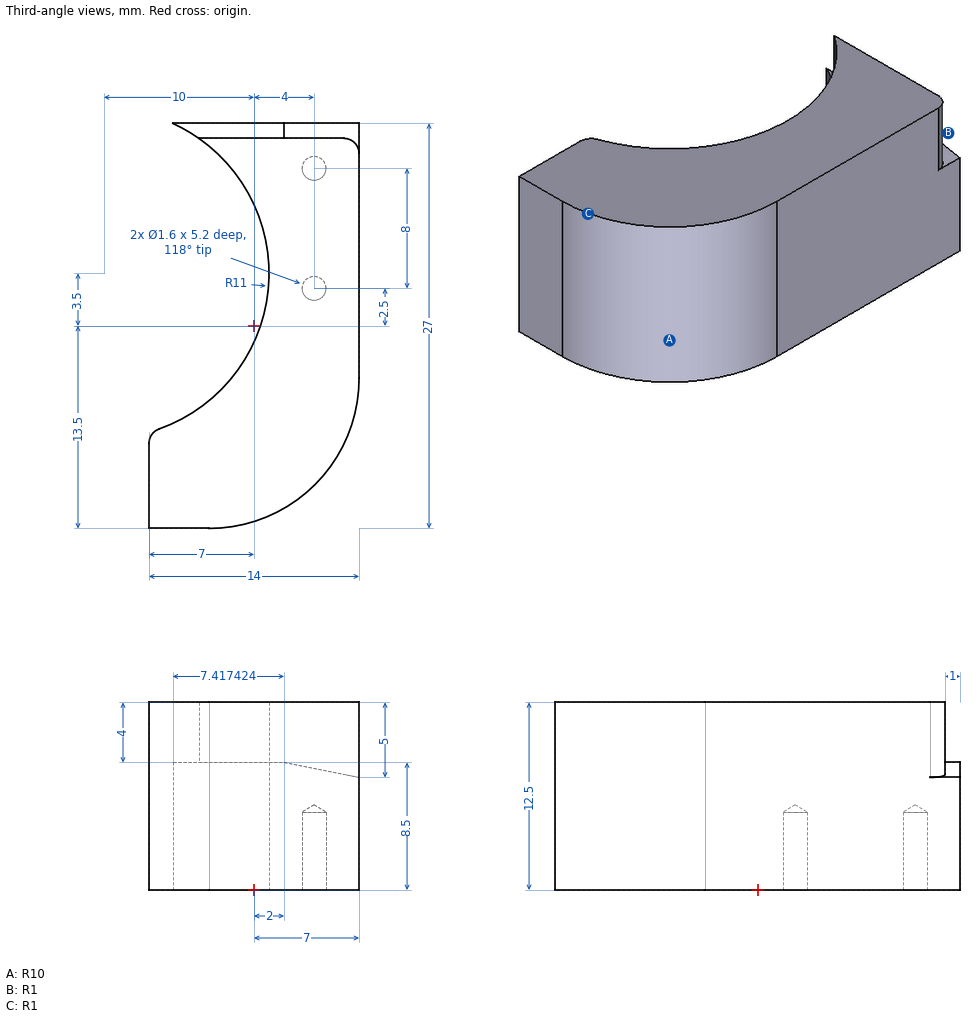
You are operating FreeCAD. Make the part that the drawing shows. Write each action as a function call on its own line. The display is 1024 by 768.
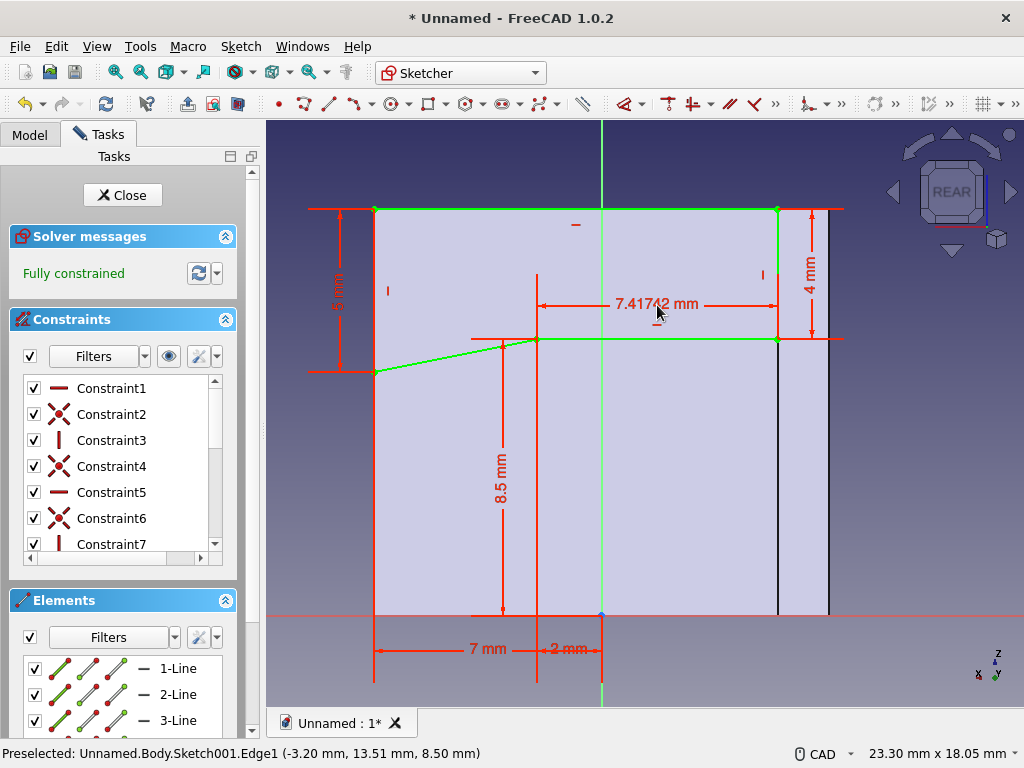
click(123, 195)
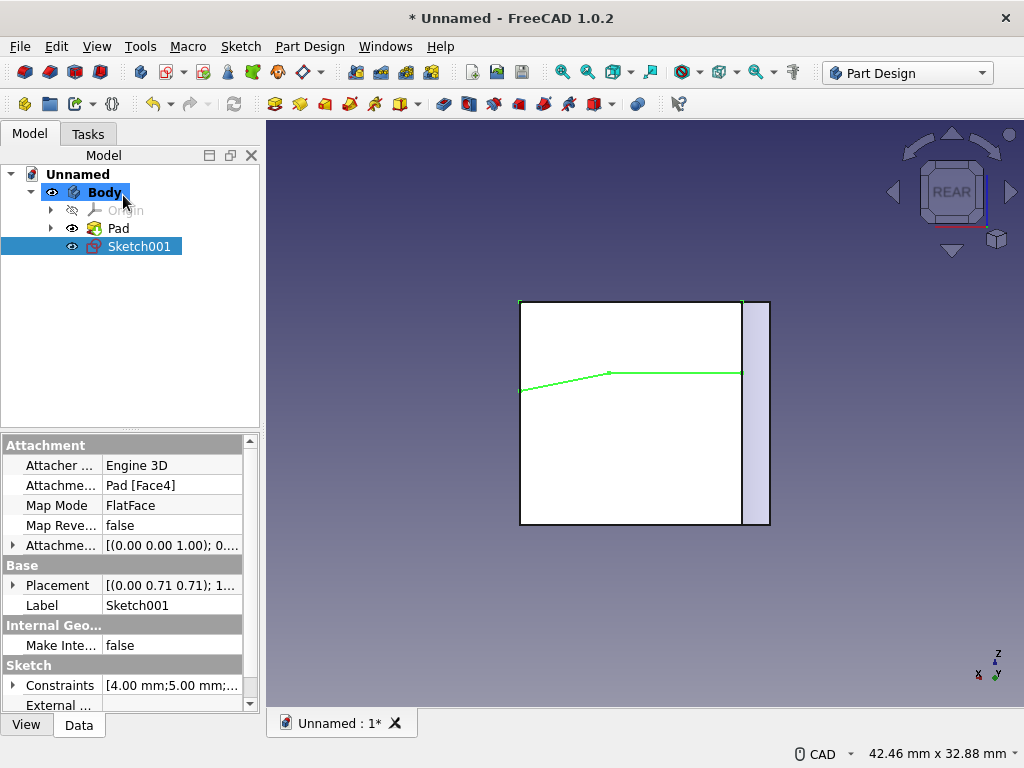
click(444, 104)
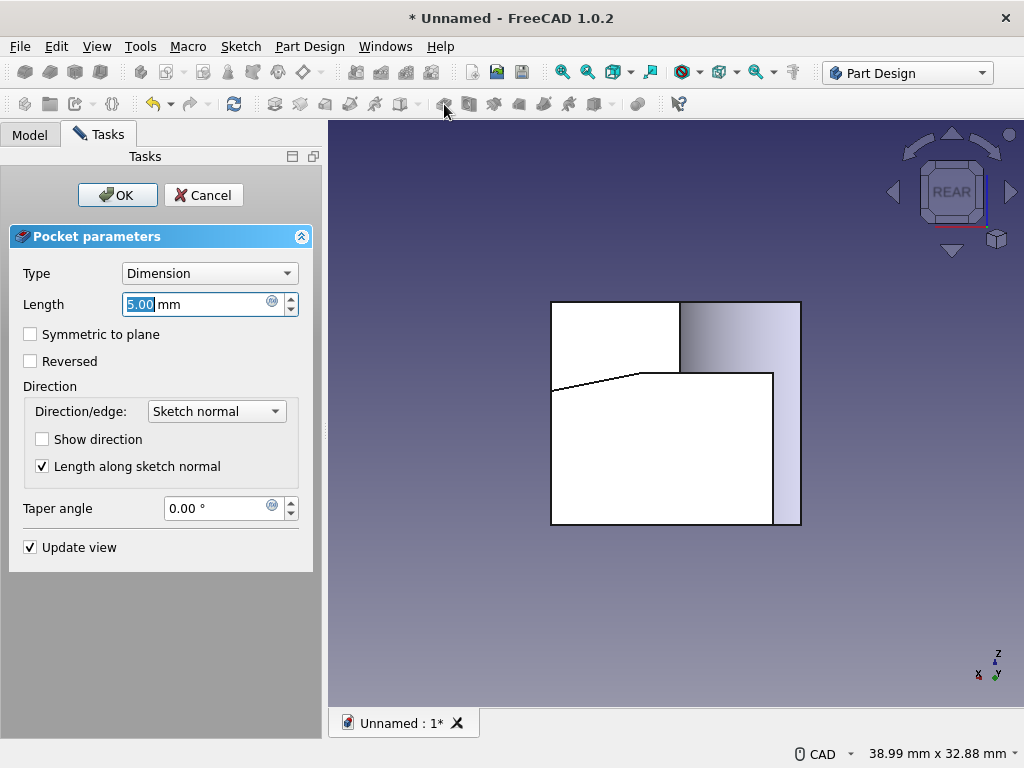
text(1)
key(Tab)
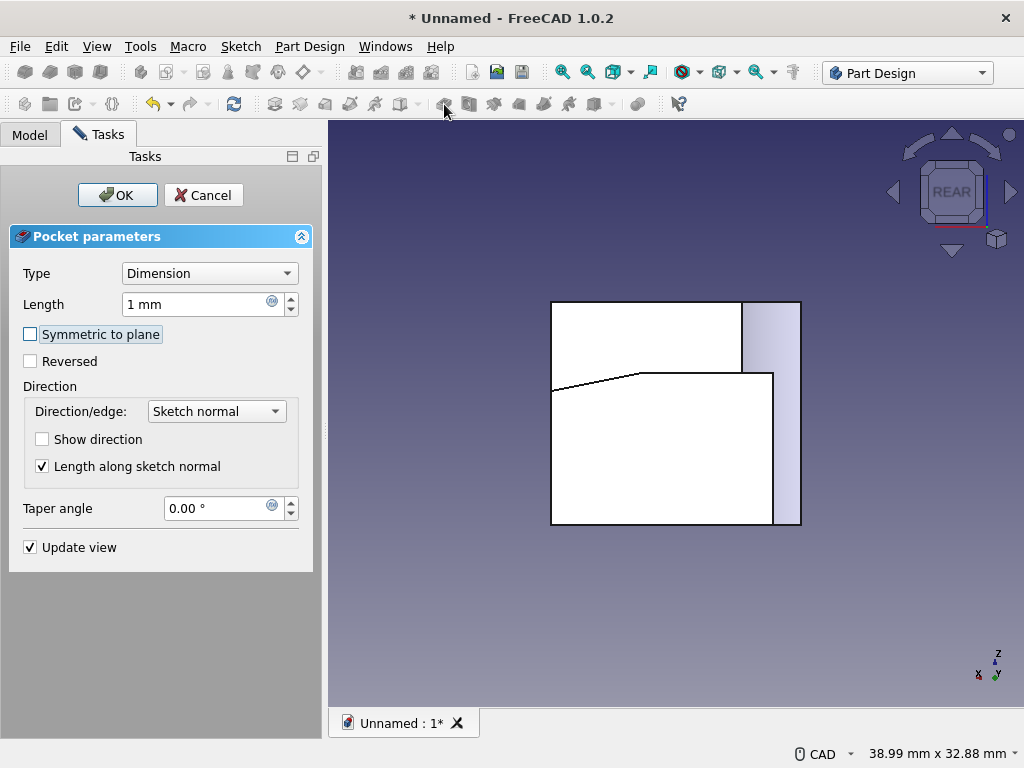
click(118, 195)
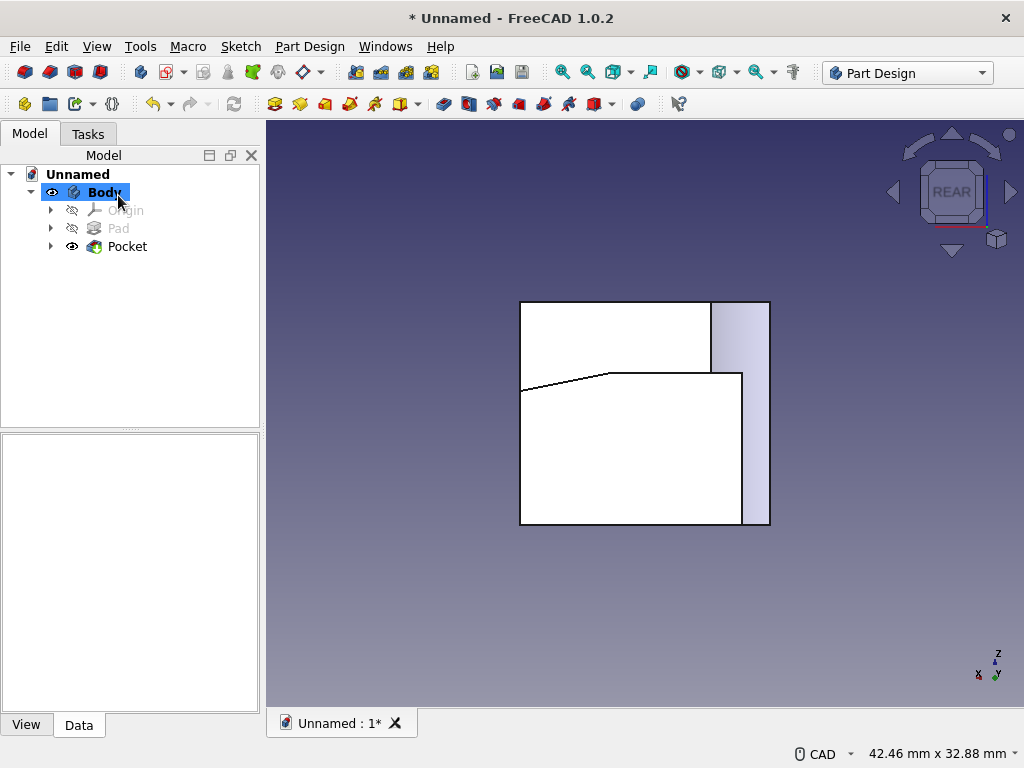
click(563, 72)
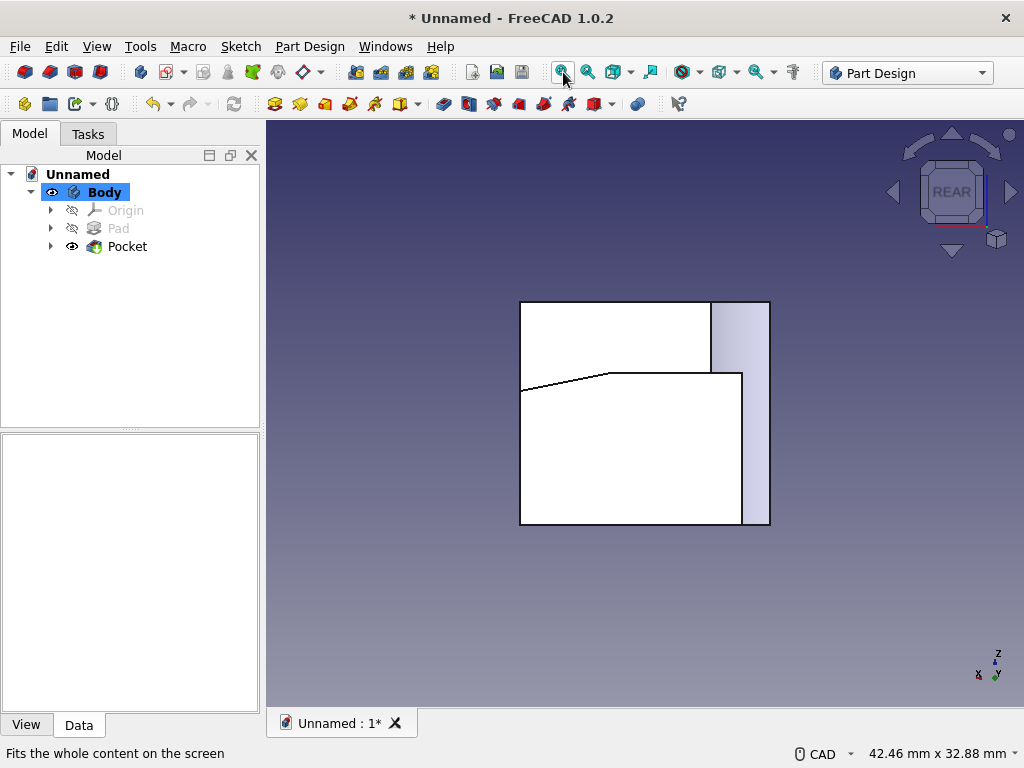
key(0)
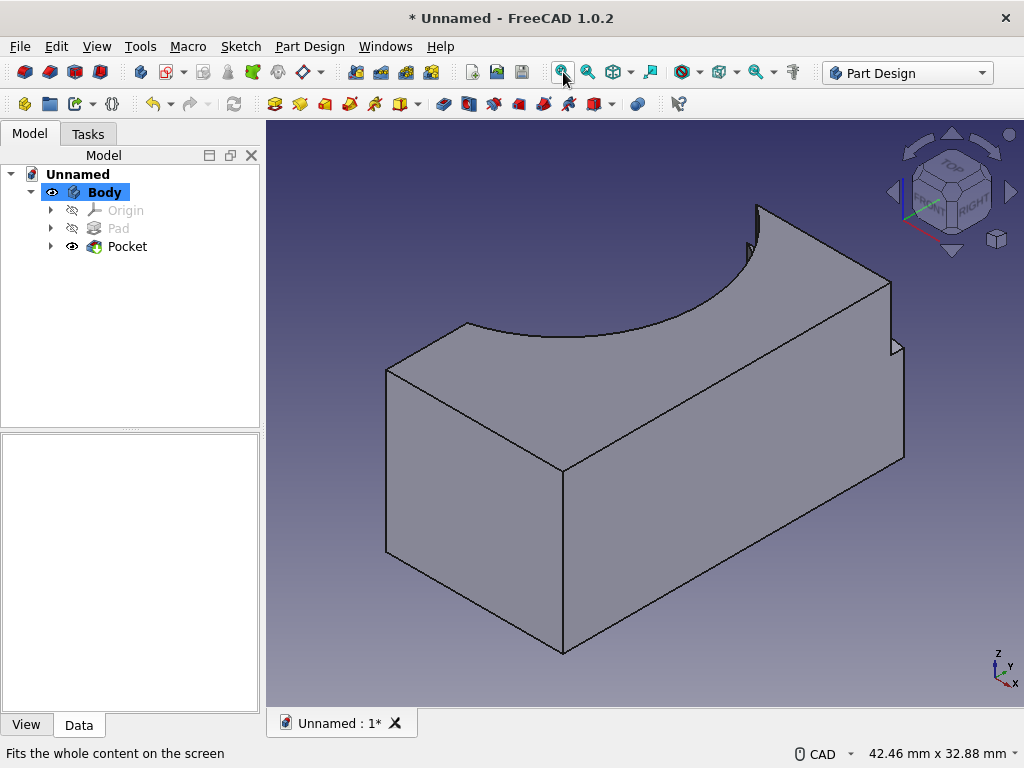
click(563, 562)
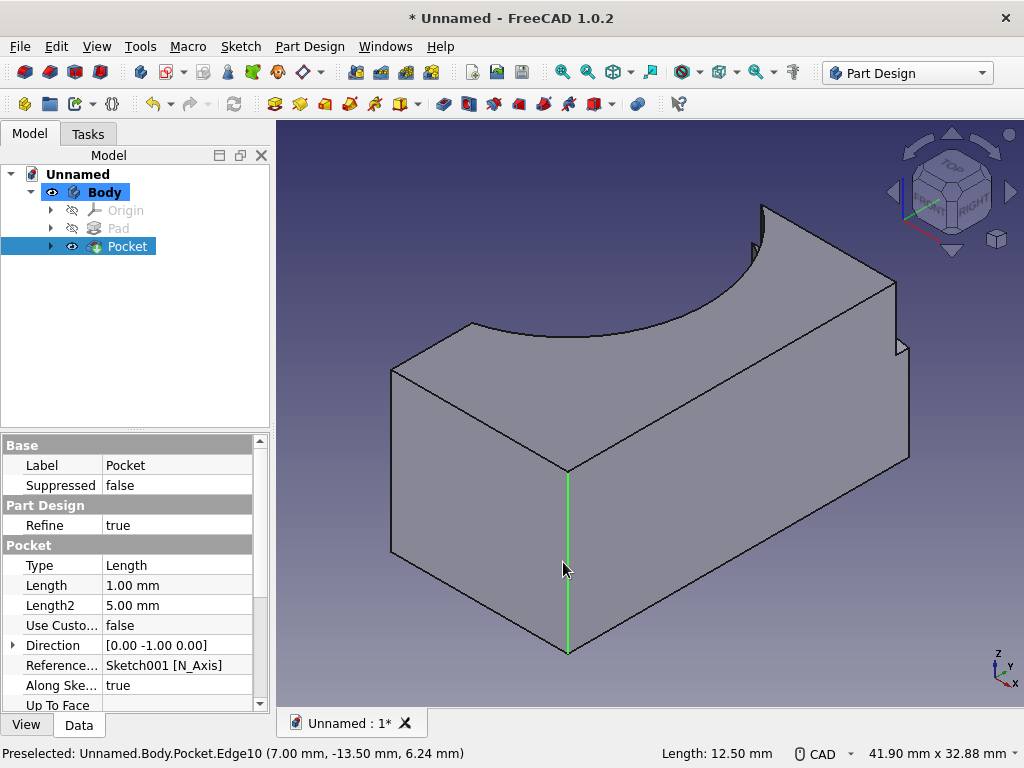
click(25, 72)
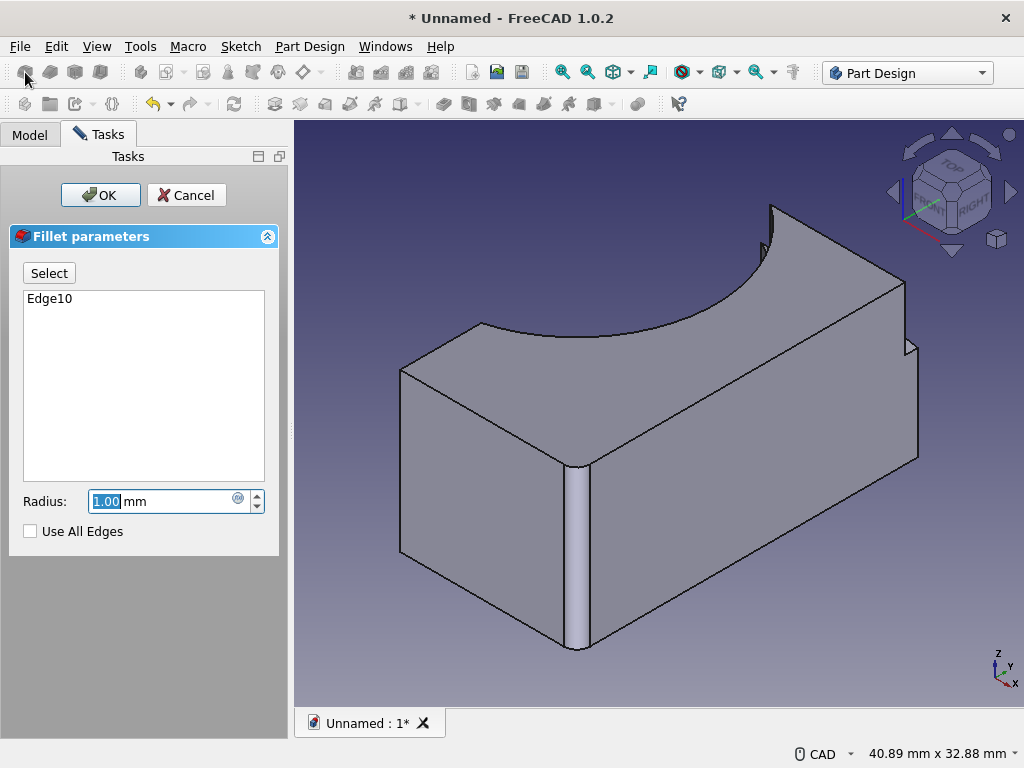
text(10)
key(Tab)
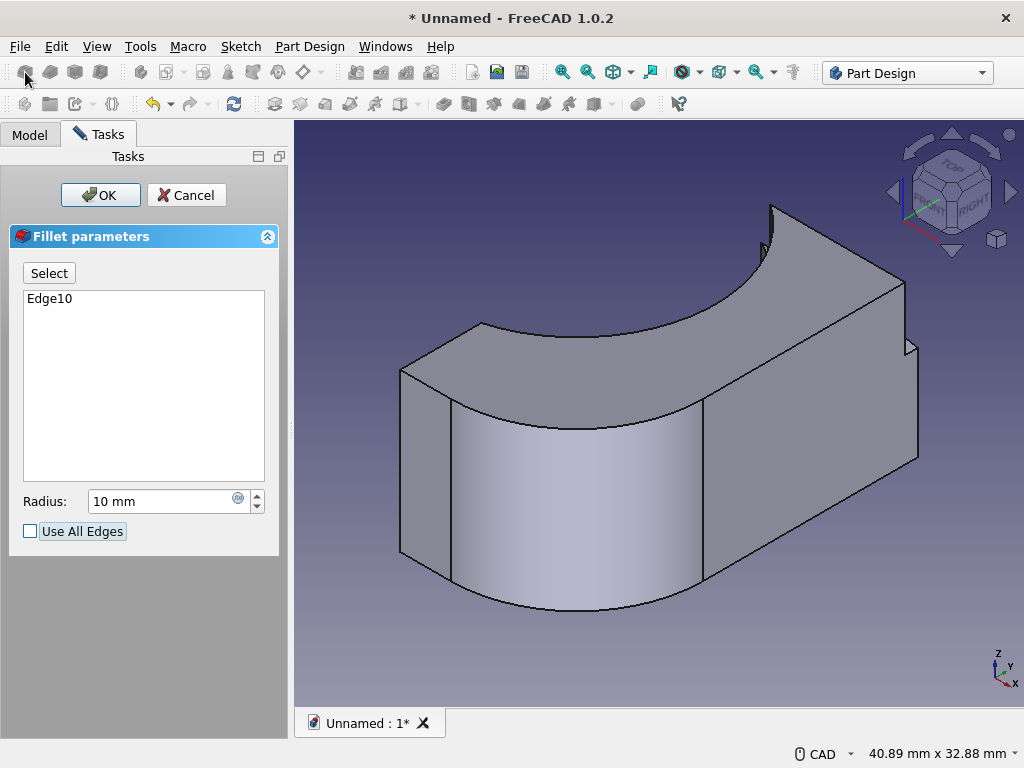
click(101, 195)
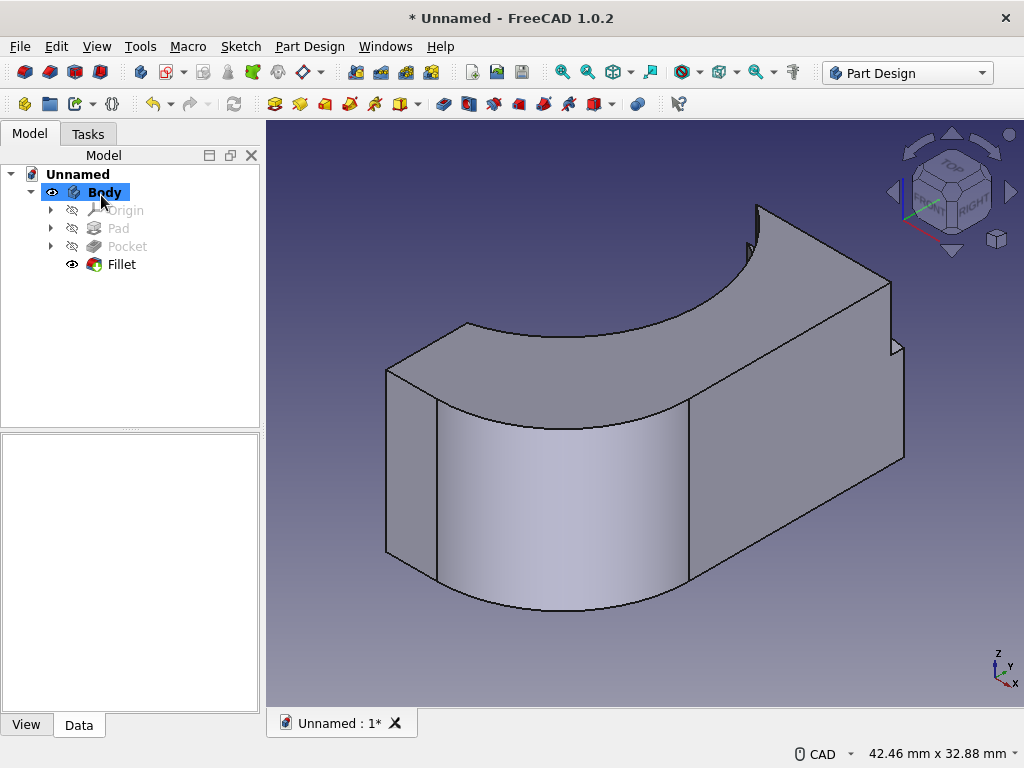
key(2)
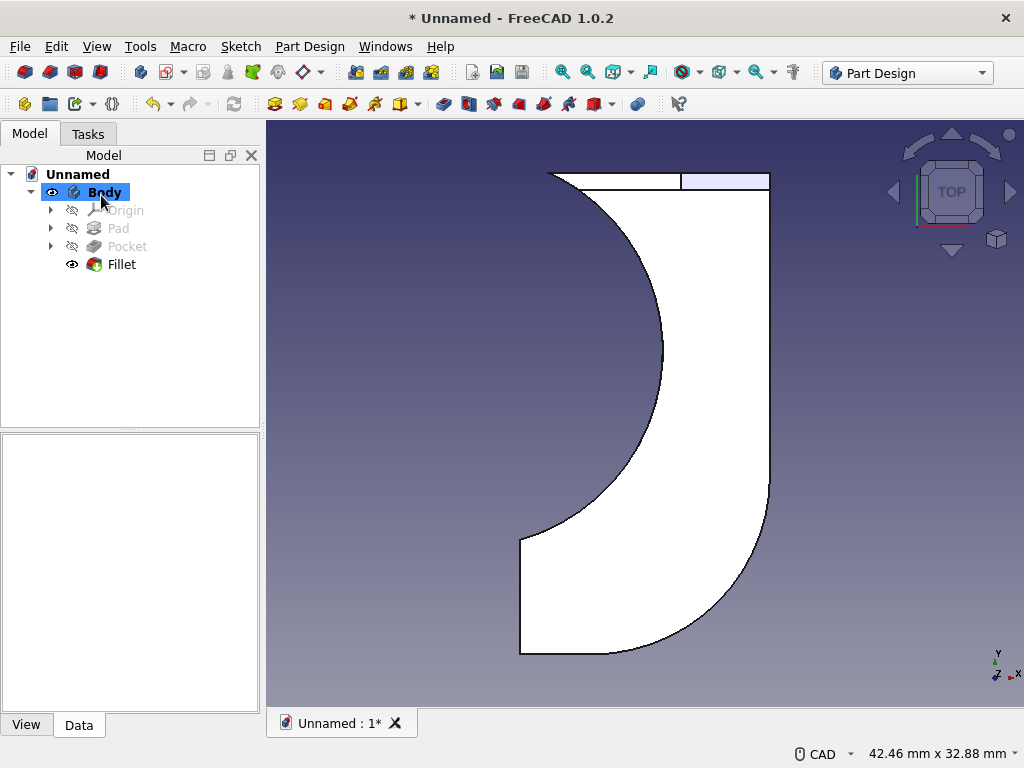
key(0)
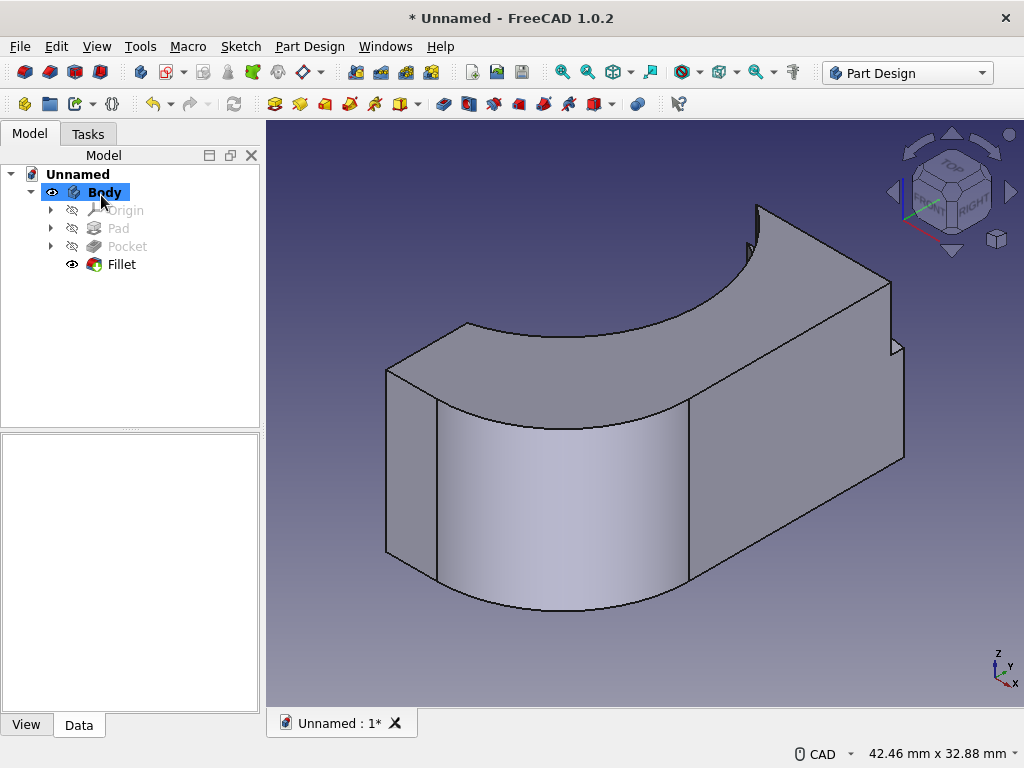
key(1)